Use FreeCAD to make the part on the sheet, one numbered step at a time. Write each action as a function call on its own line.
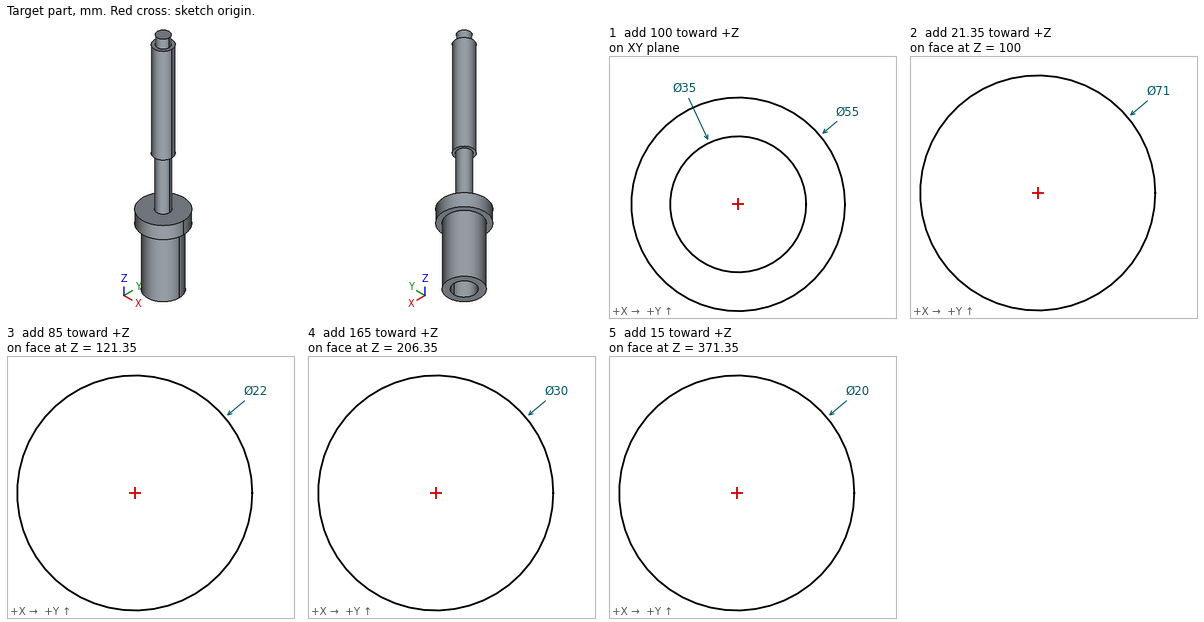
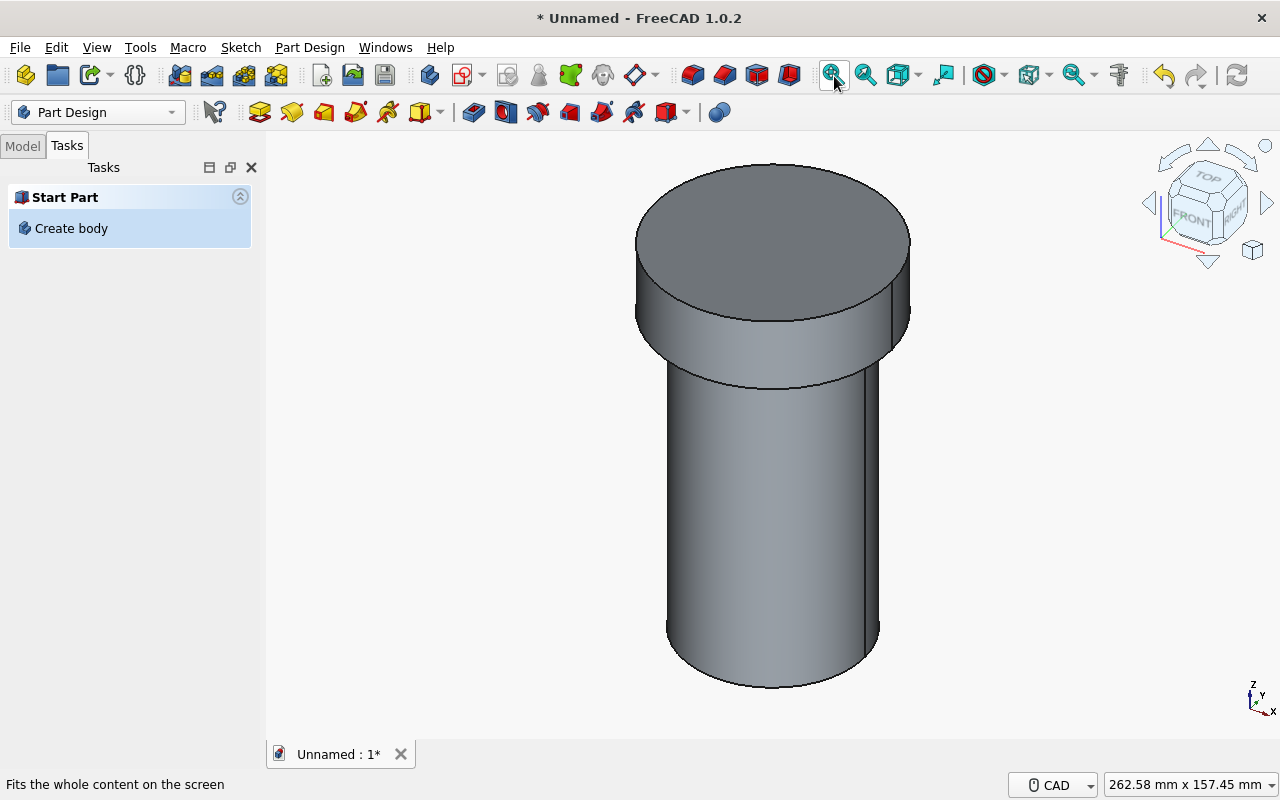
click(773, 242)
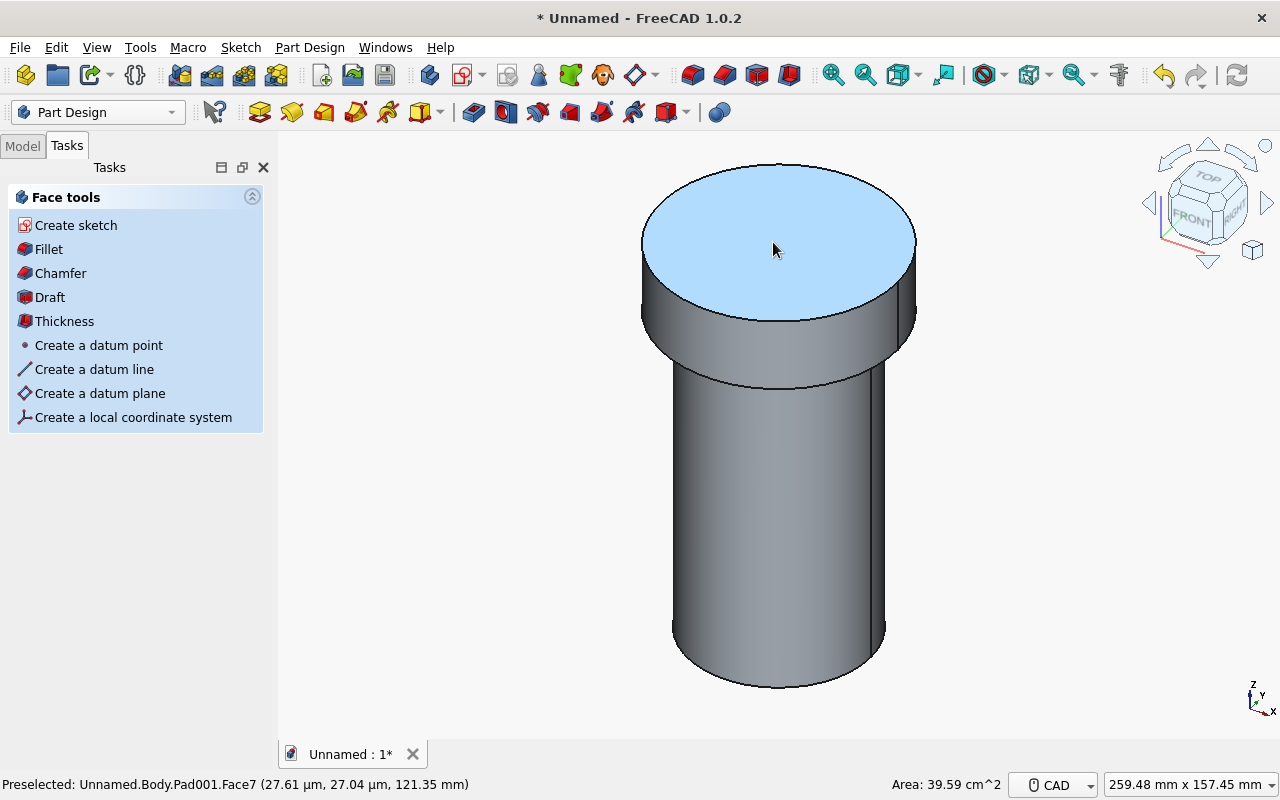
click(462, 76)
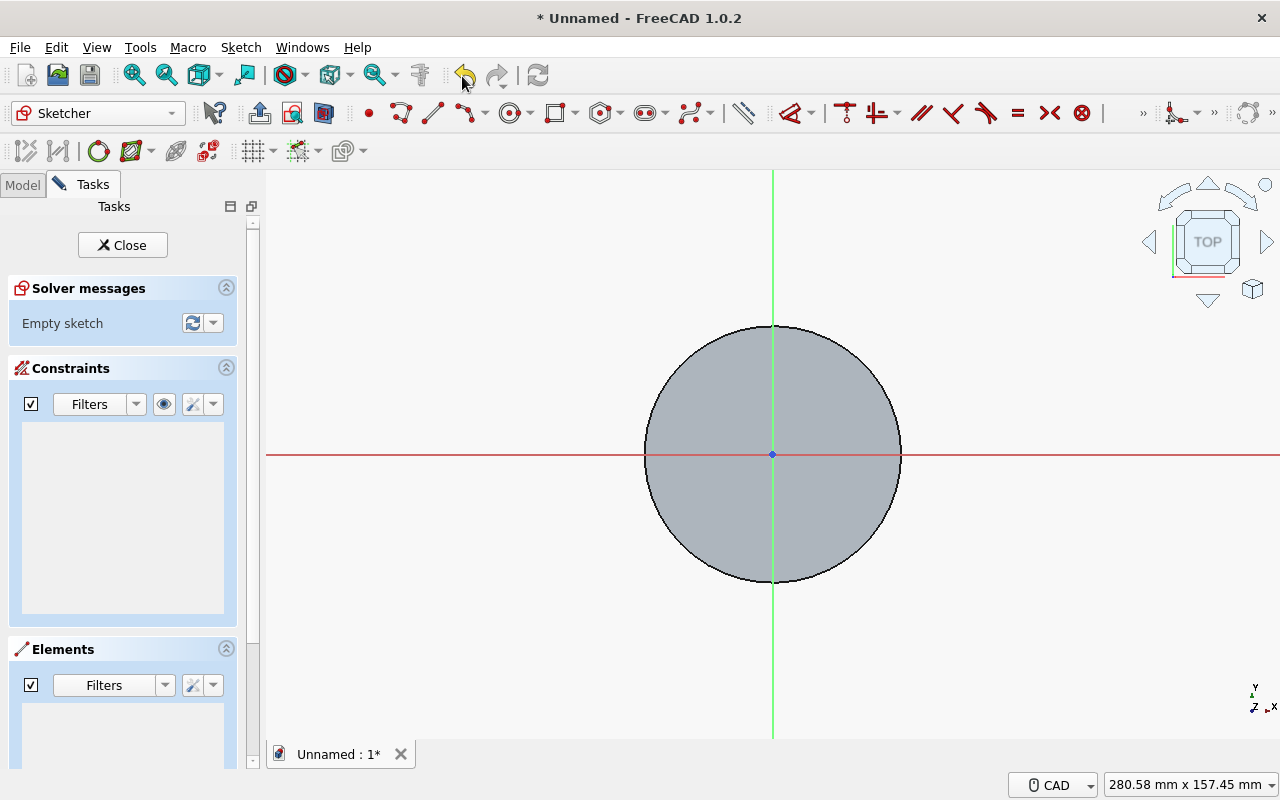
scroll(790, 454, up, 8)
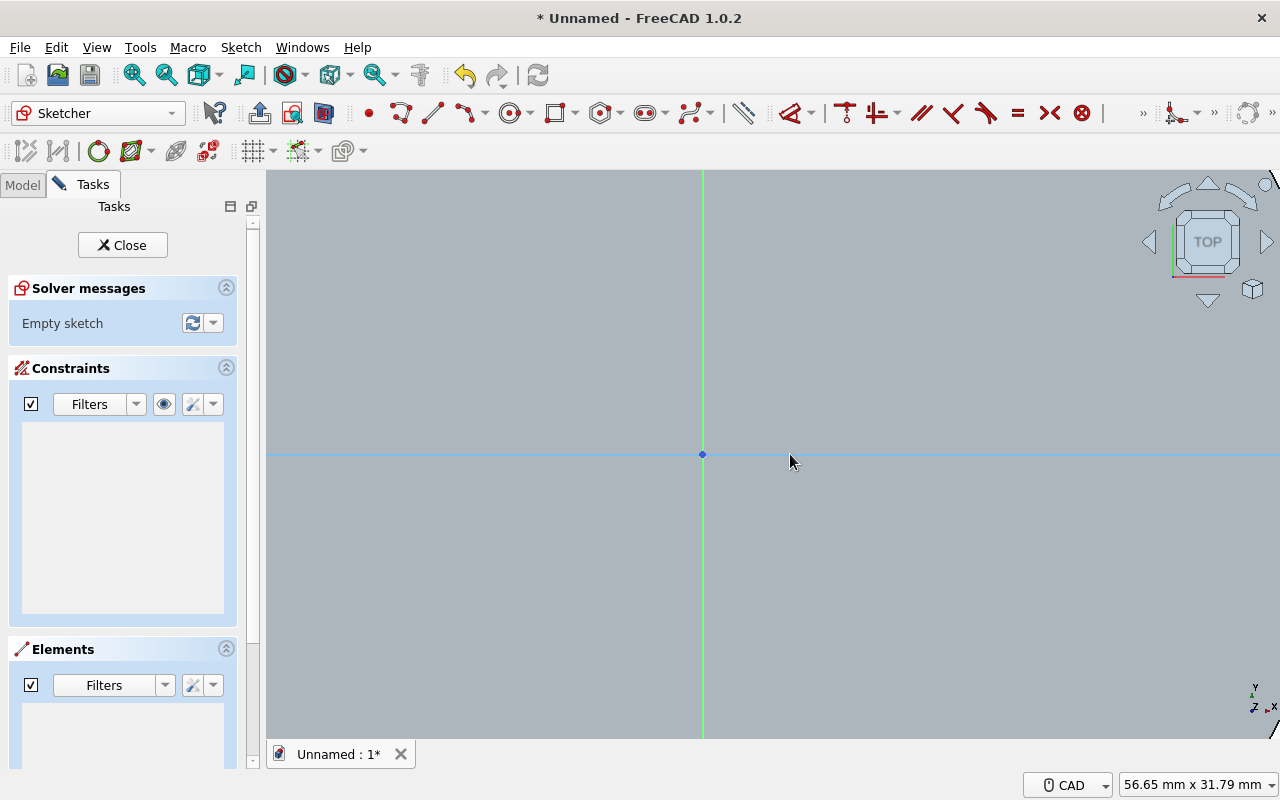
key(g)
key(c)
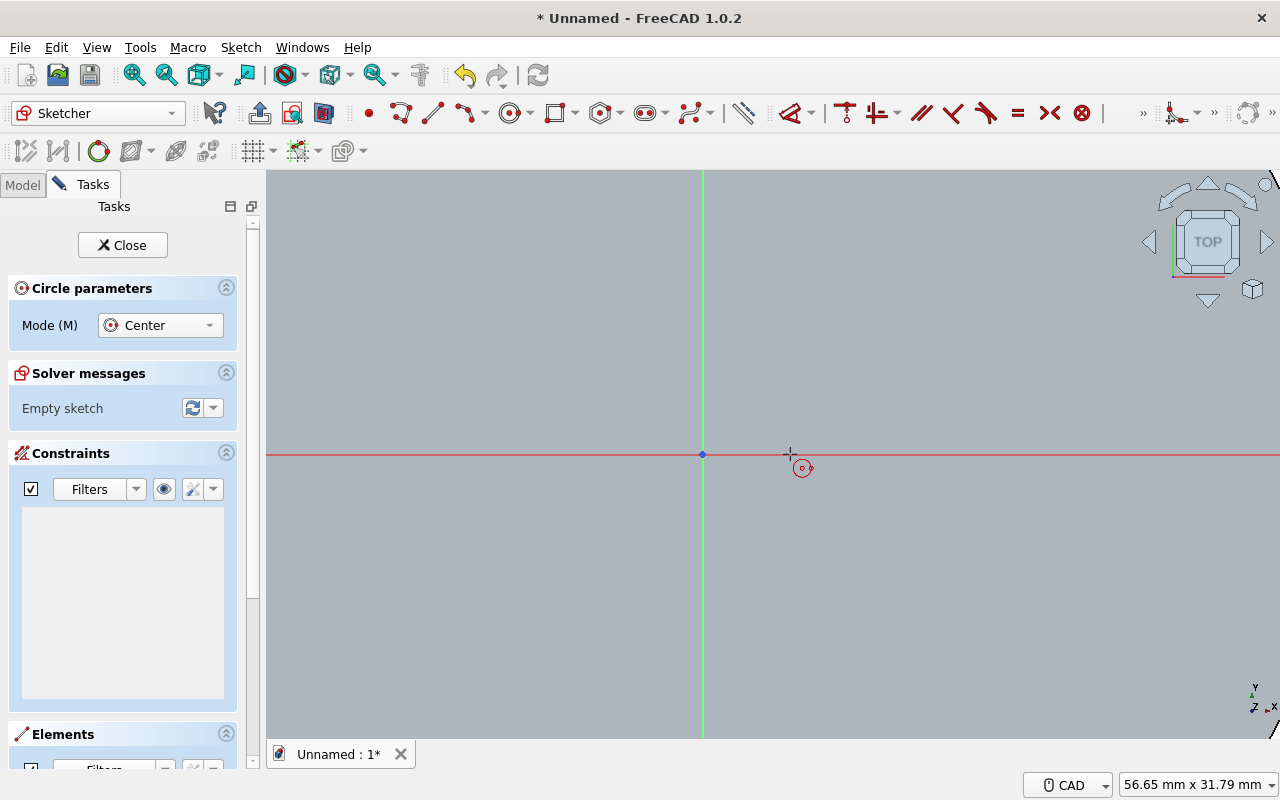
click(703, 454)
click(842, 315)
key(Escape)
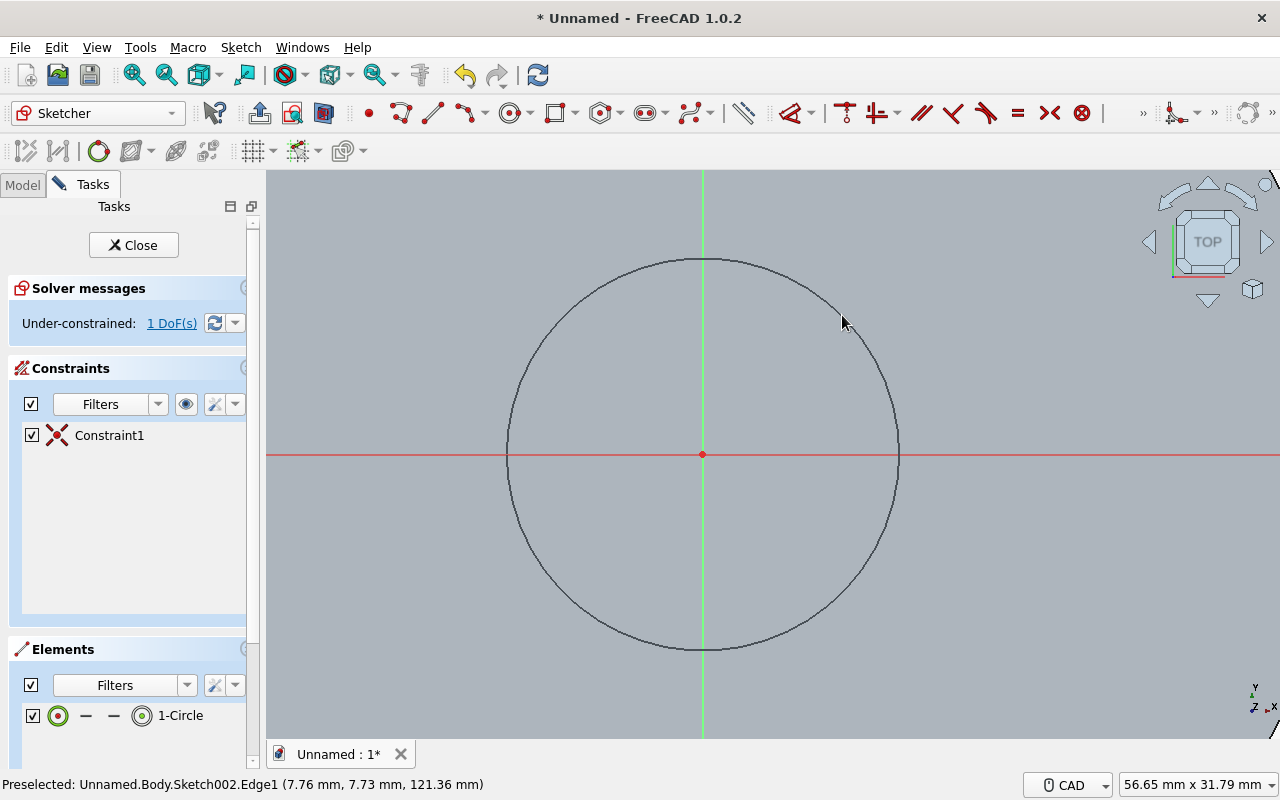
click(841, 315)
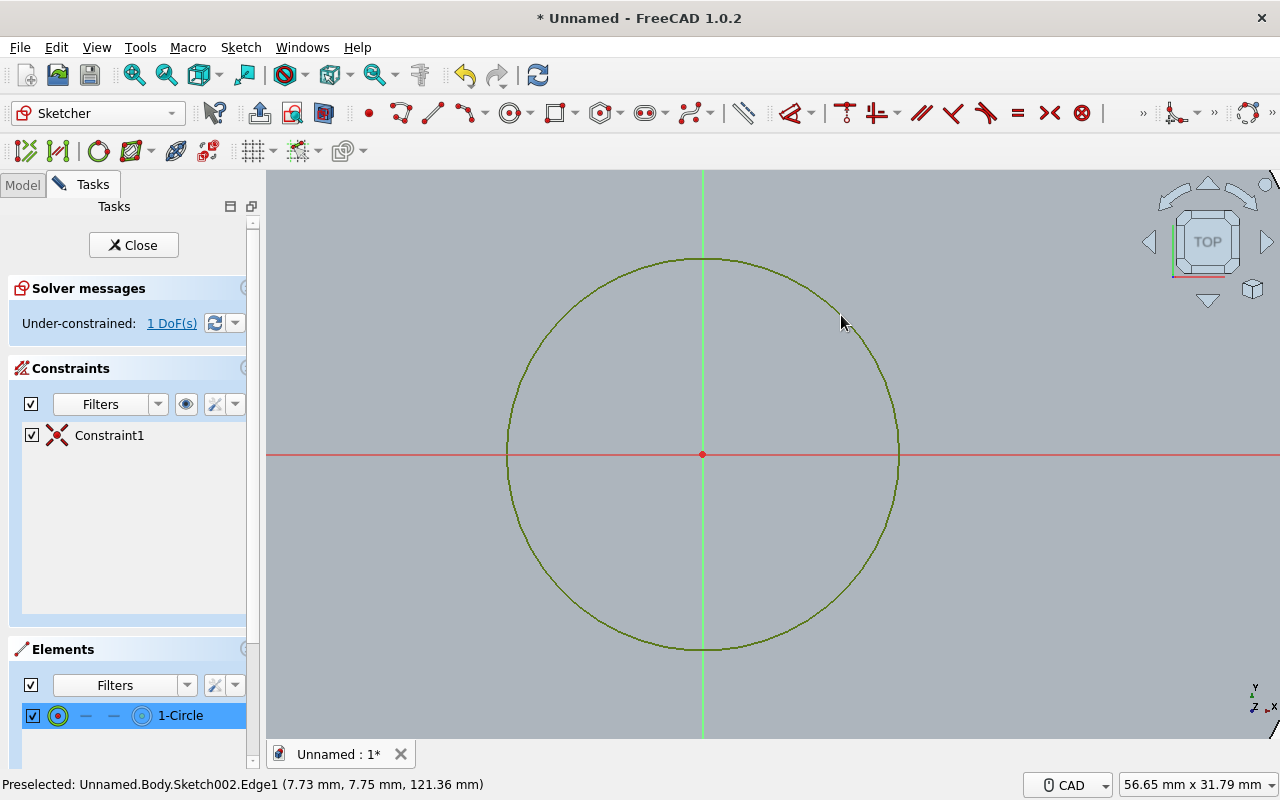
key(k)
key(o)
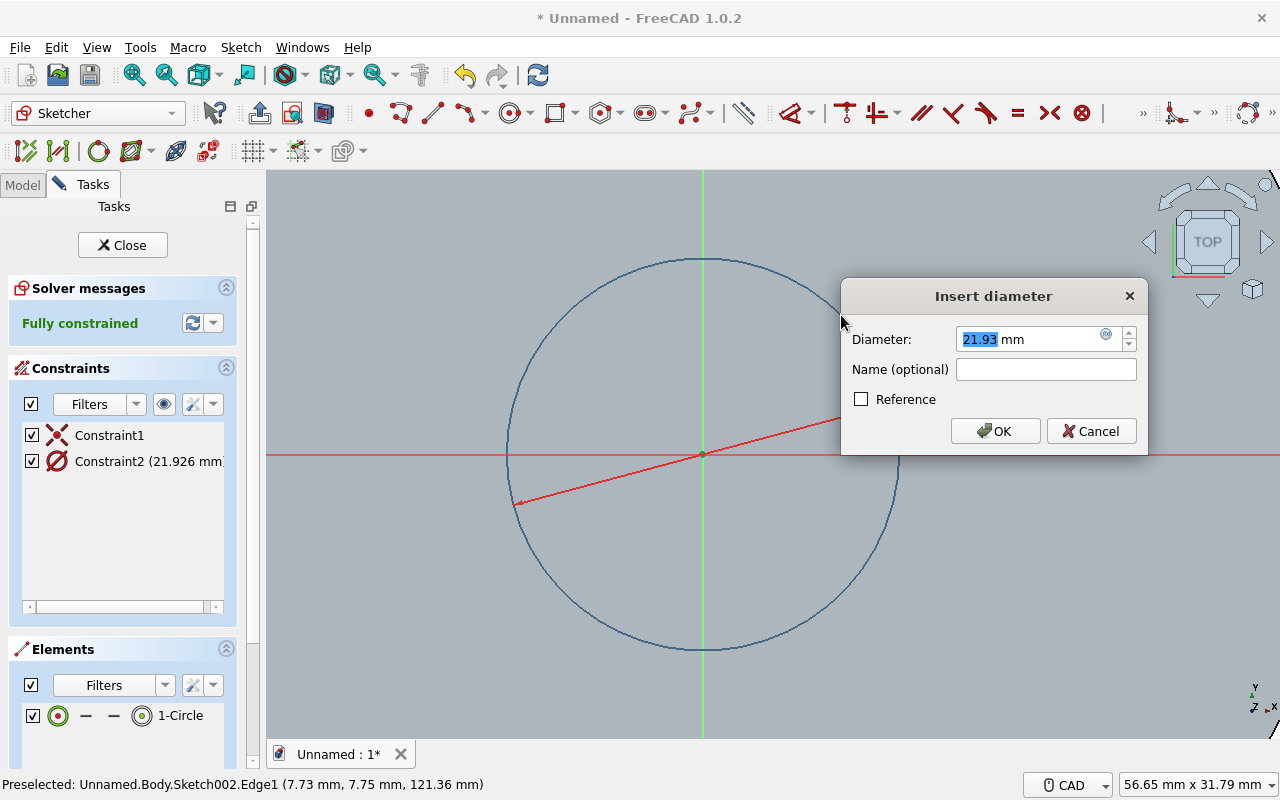
text(22)
key(Return)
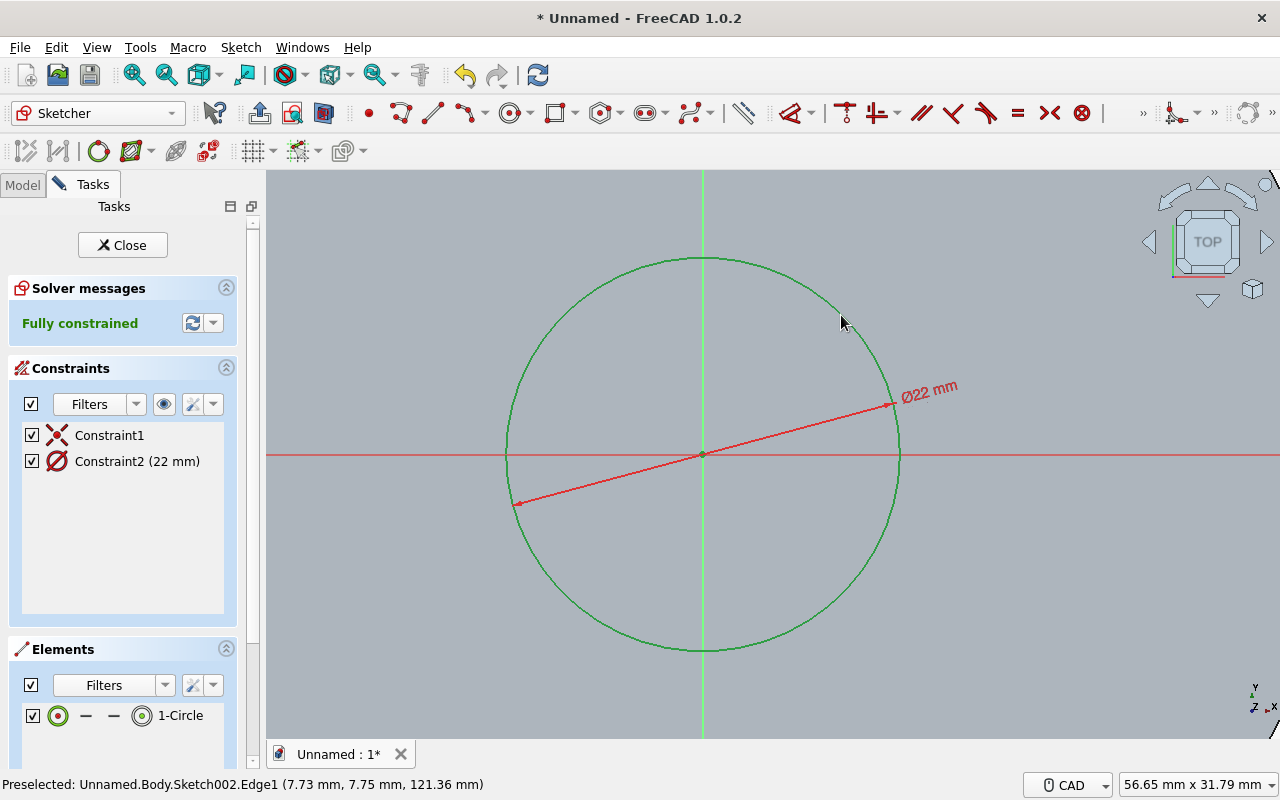
click(123, 245)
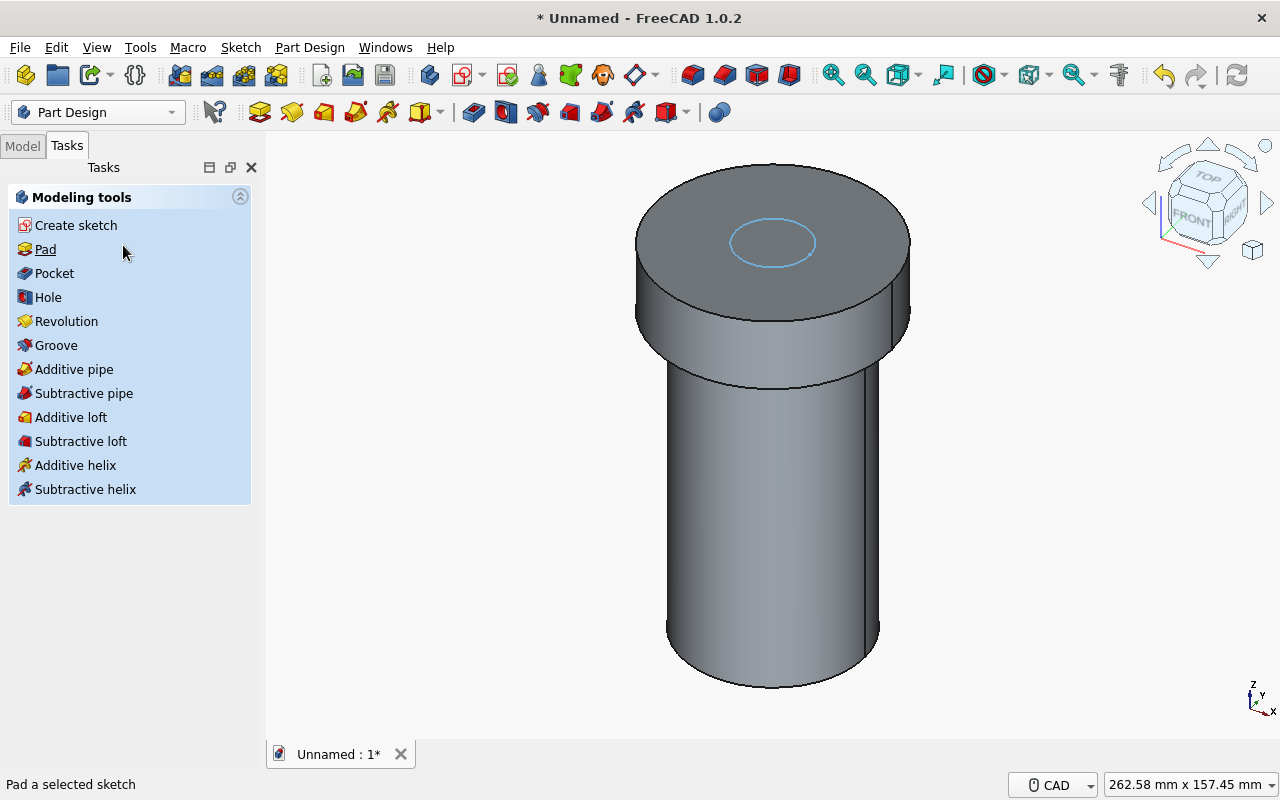
click(260, 112)